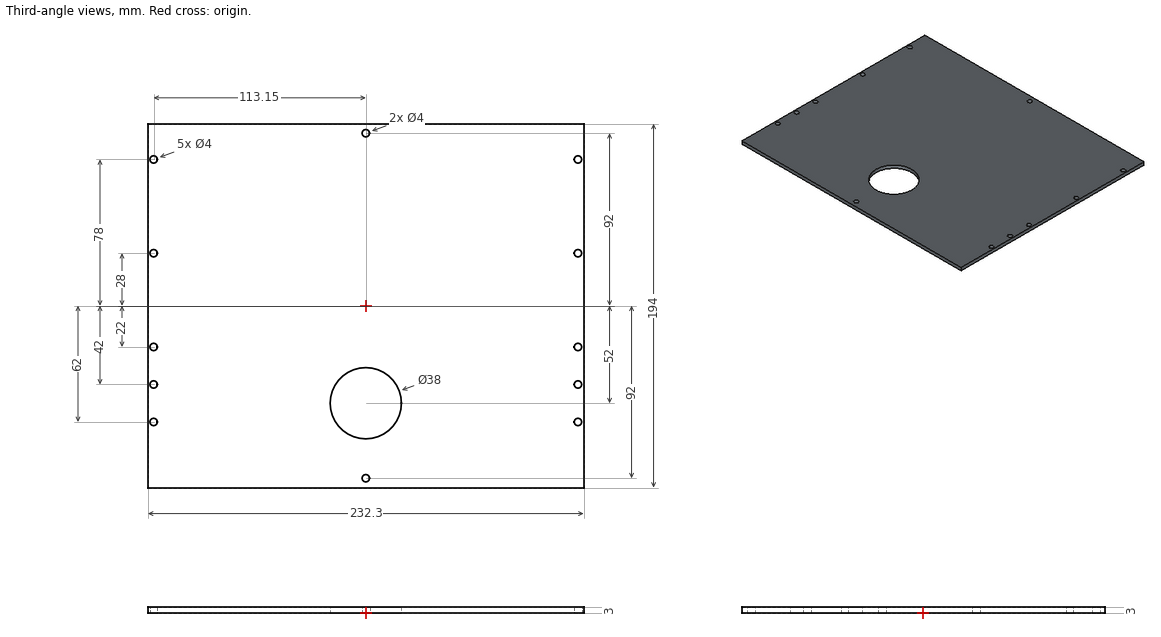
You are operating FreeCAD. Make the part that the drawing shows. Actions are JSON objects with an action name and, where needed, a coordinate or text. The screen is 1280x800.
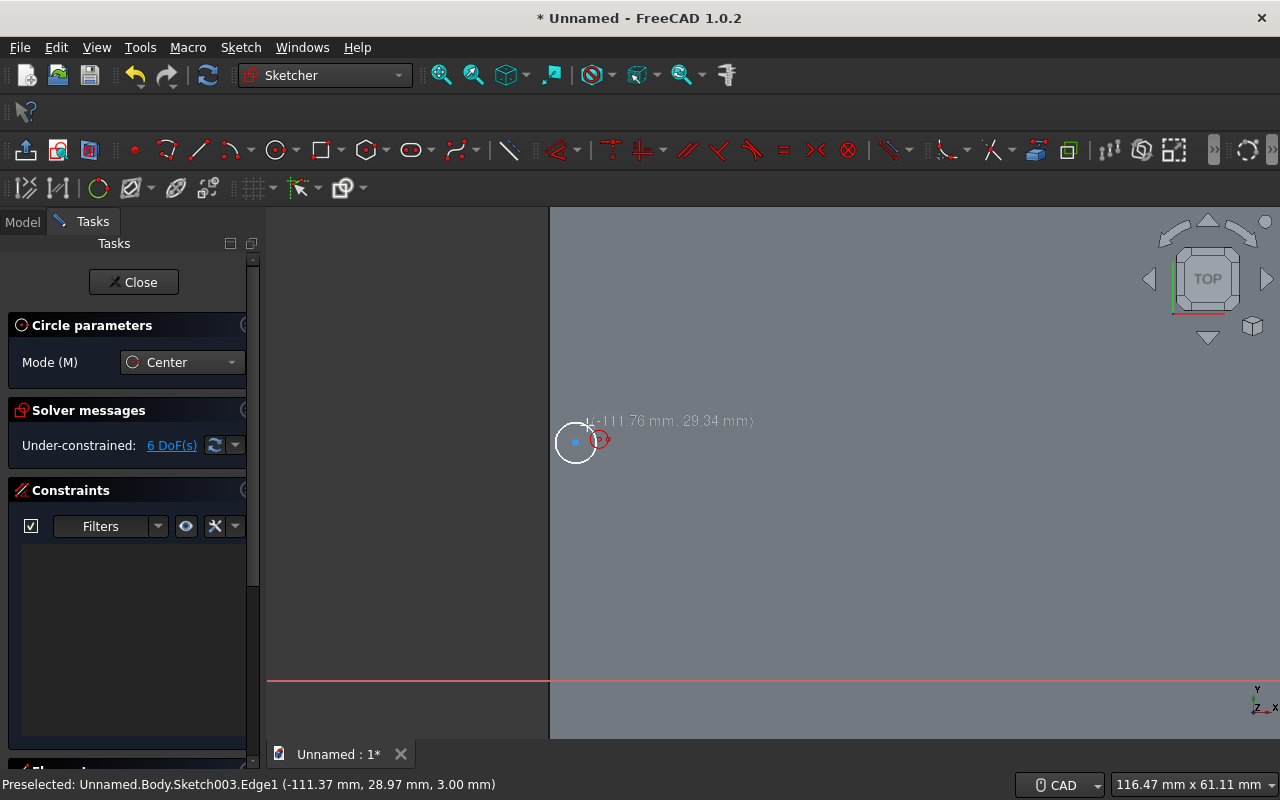
{"action": "scroll", "coordinate": [589, 428], "scroll_direction": "down", "scroll_amount": 7}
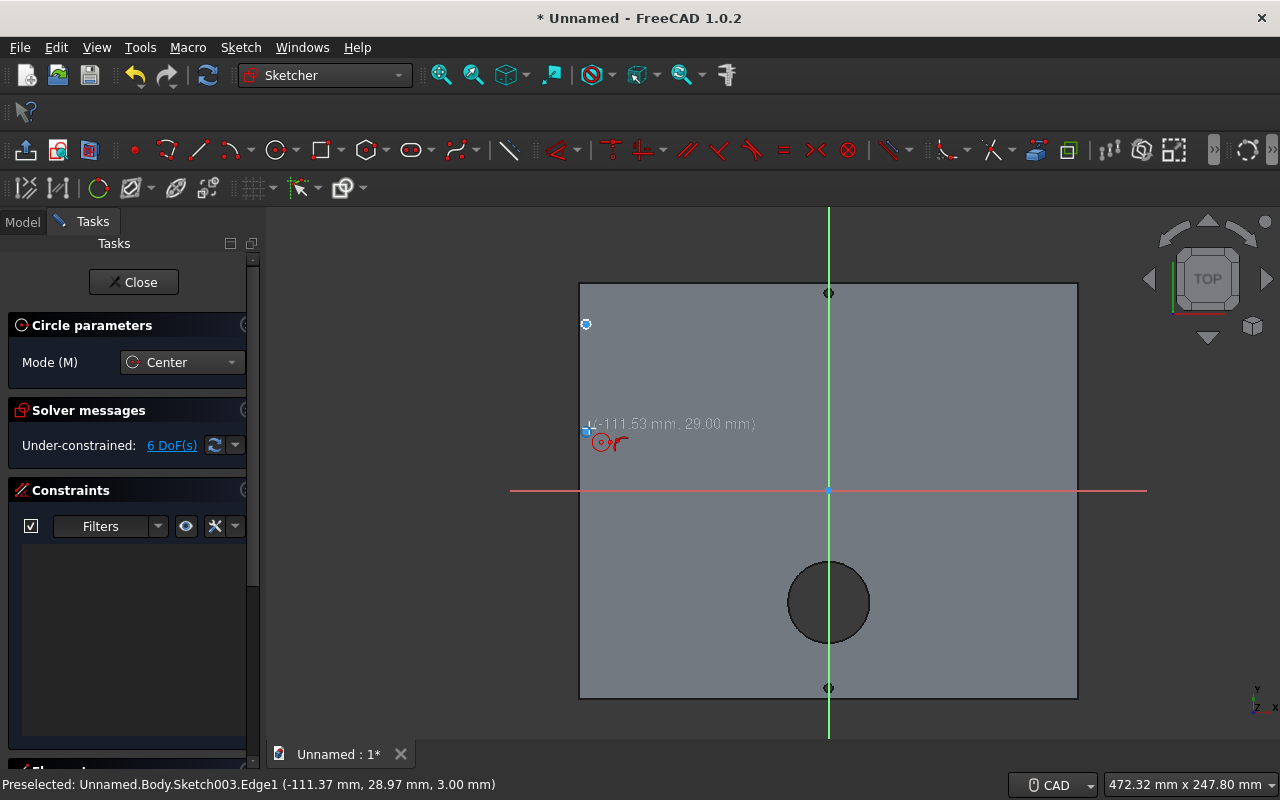
{"action": "scroll", "coordinate": [586, 538], "scroll_direction": "up", "scroll_amount": 9}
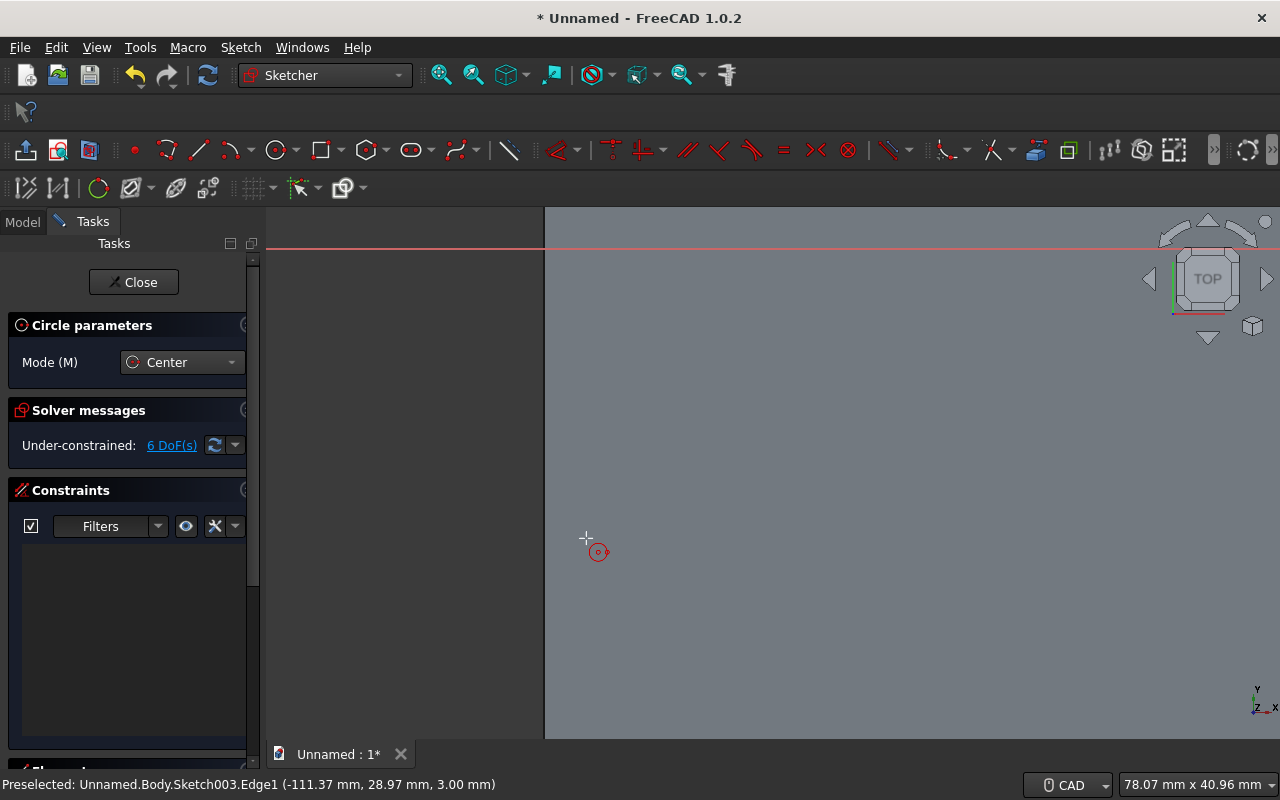
{"action": "scroll", "coordinate": [586, 538], "scroll_direction": "down", "scroll_amount": 9}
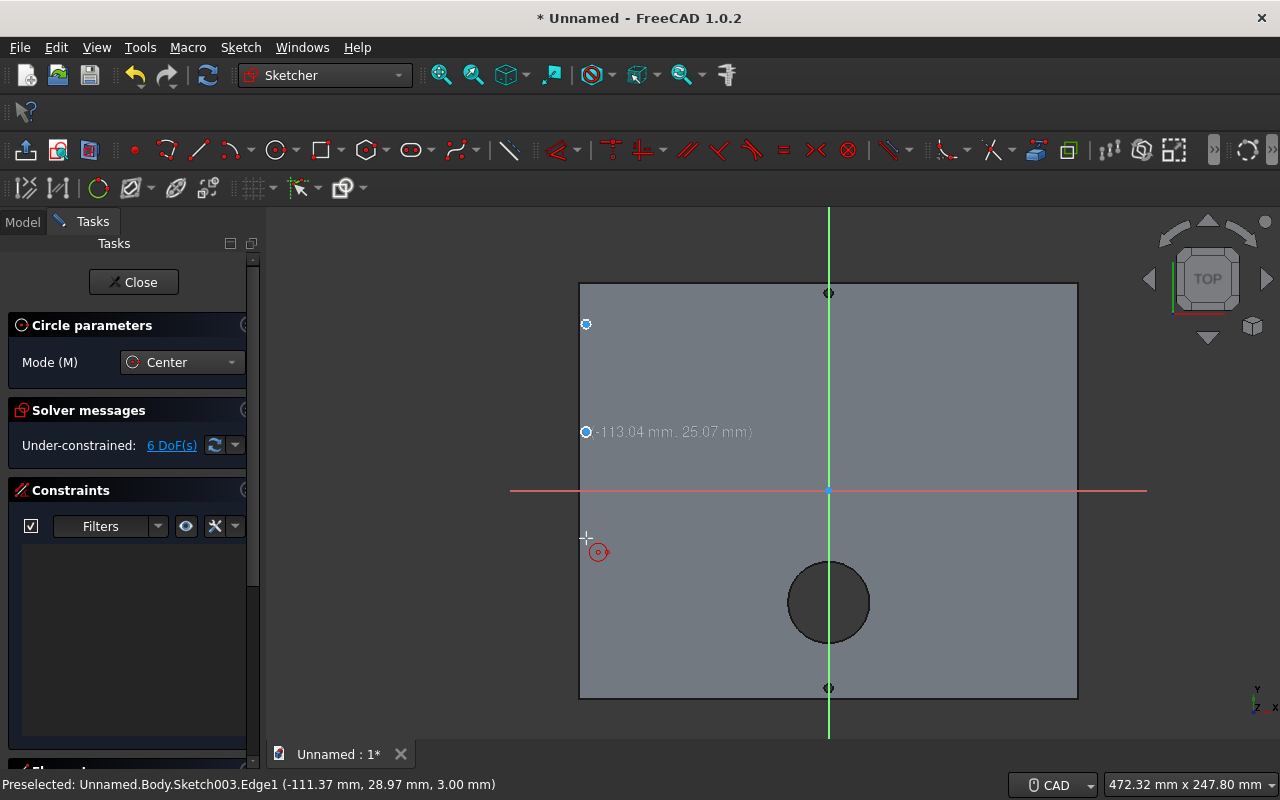
{"action": "left_click", "coordinate": [586, 538]}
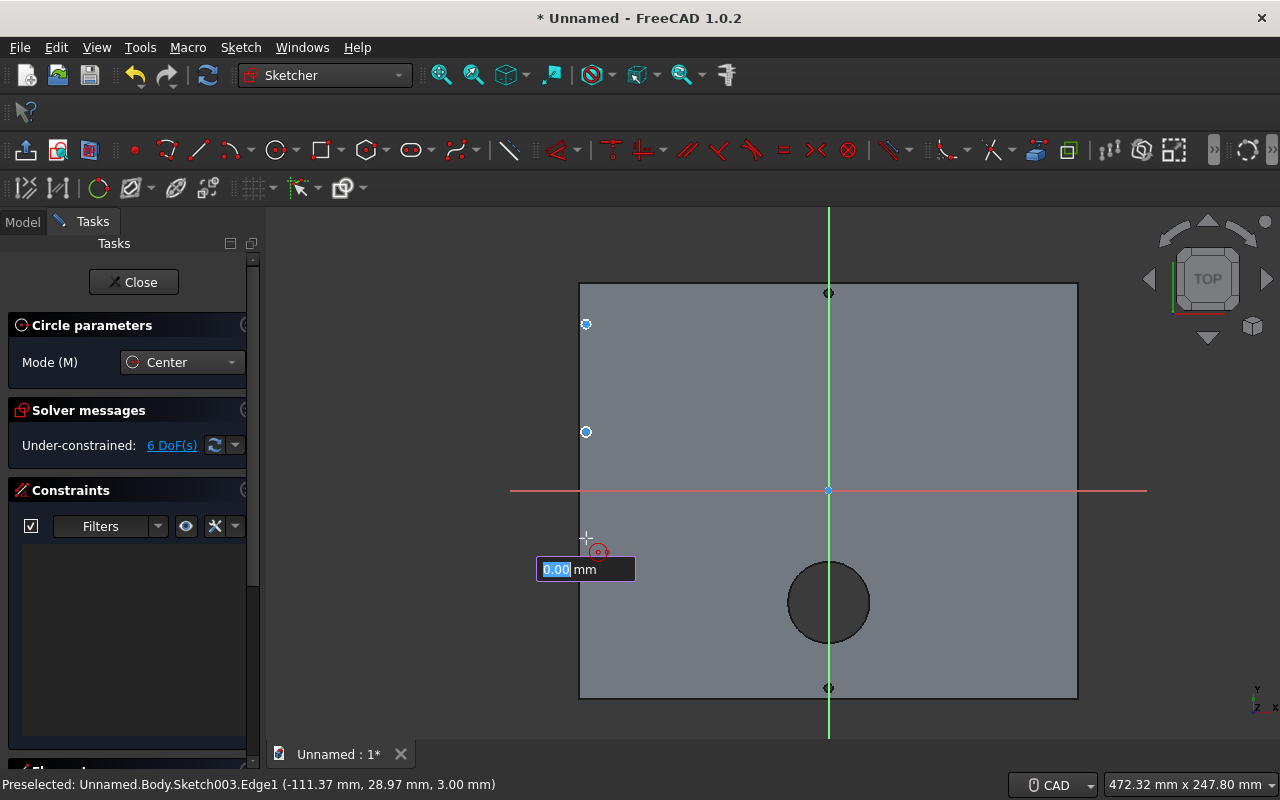
{"action": "scroll", "coordinate": [589, 535], "scroll_direction": "up", "scroll_amount": 7}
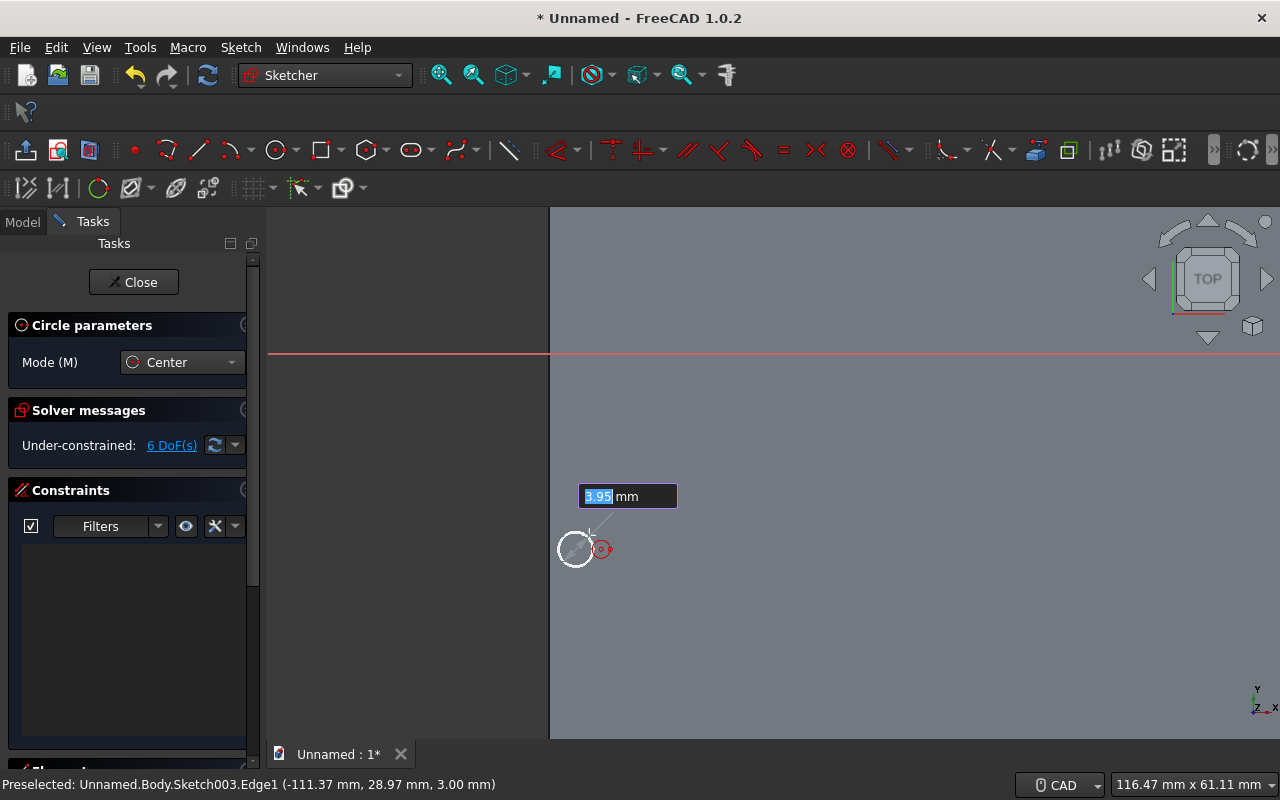
{"action": "left_click", "coordinate": [587, 533]}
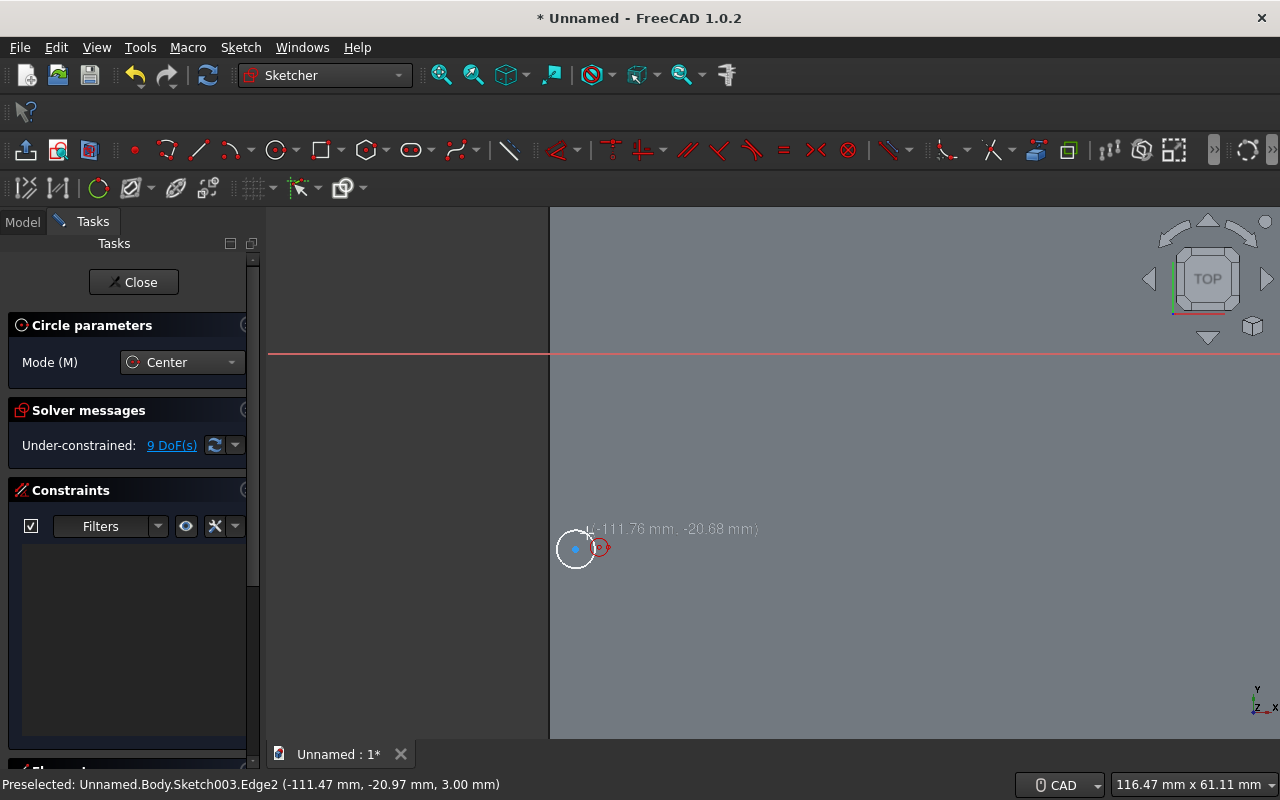
{"action": "scroll", "coordinate": [589, 535], "scroll_direction": "down", "scroll_amount": 7}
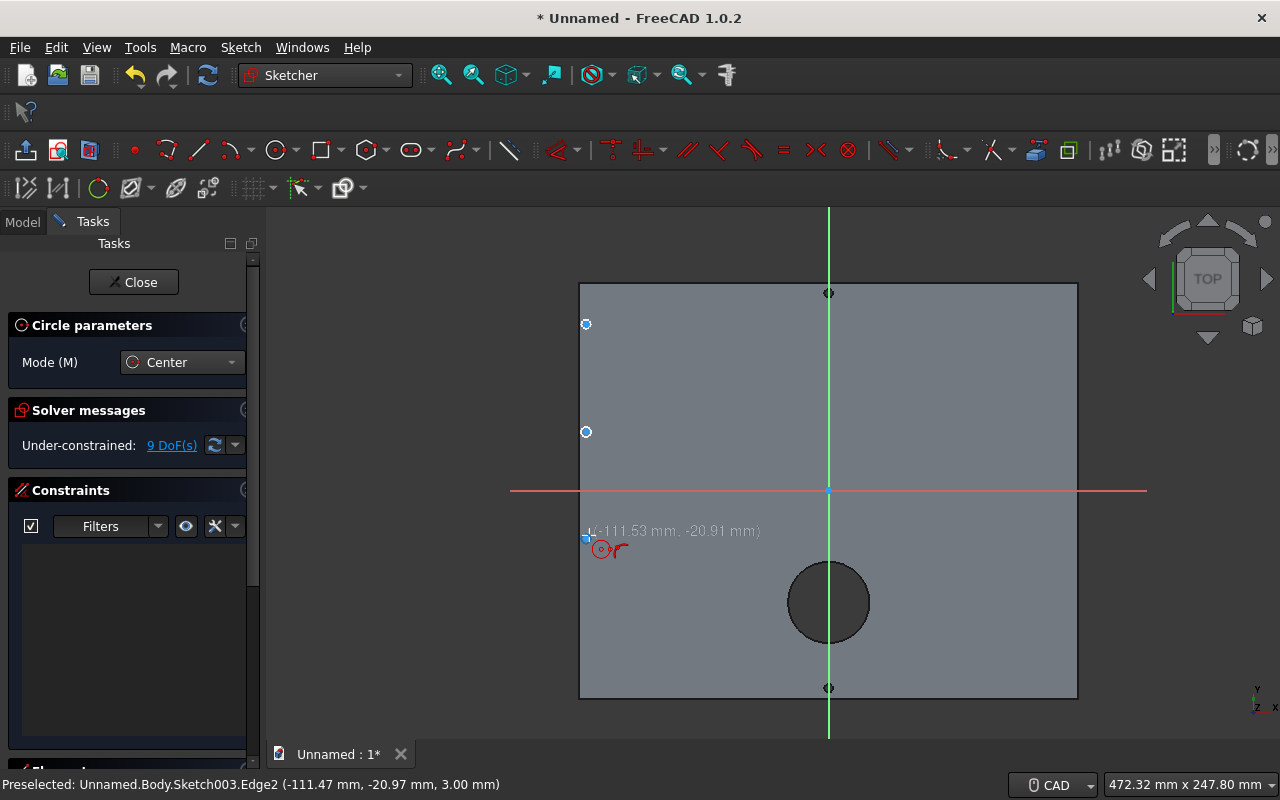
{"action": "scroll", "coordinate": [586, 581], "scroll_direction": "up", "scroll_amount": 9}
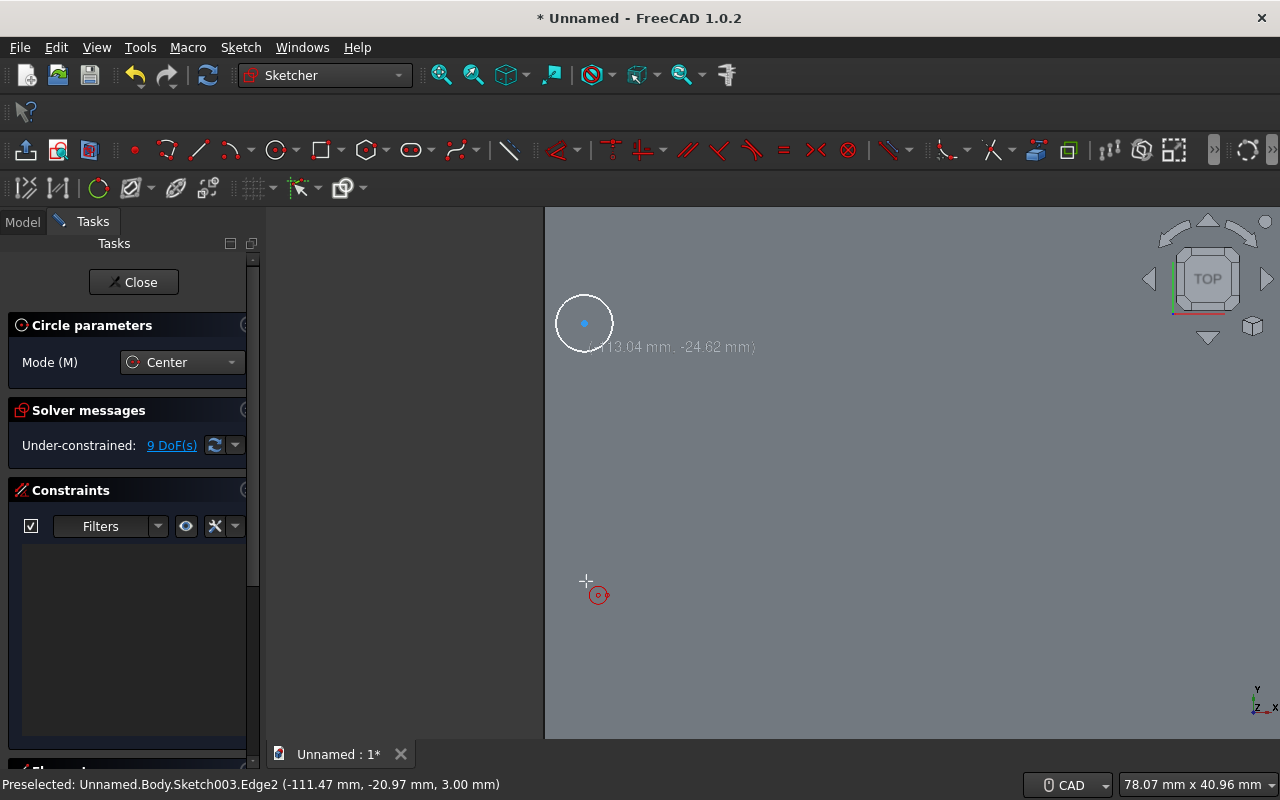
{"action": "scroll", "coordinate": [586, 581], "scroll_direction": "down", "scroll_amount": 9}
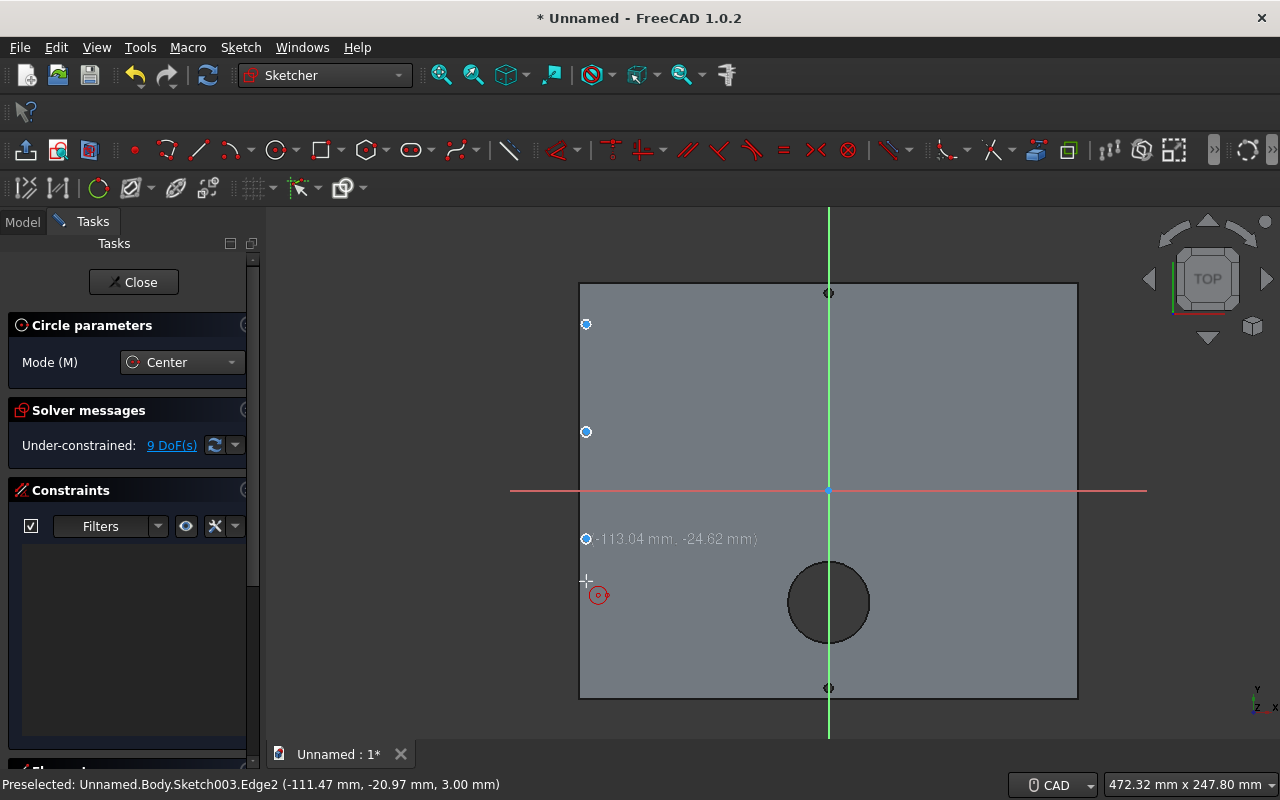
{"action": "left_click", "coordinate": [586, 581]}